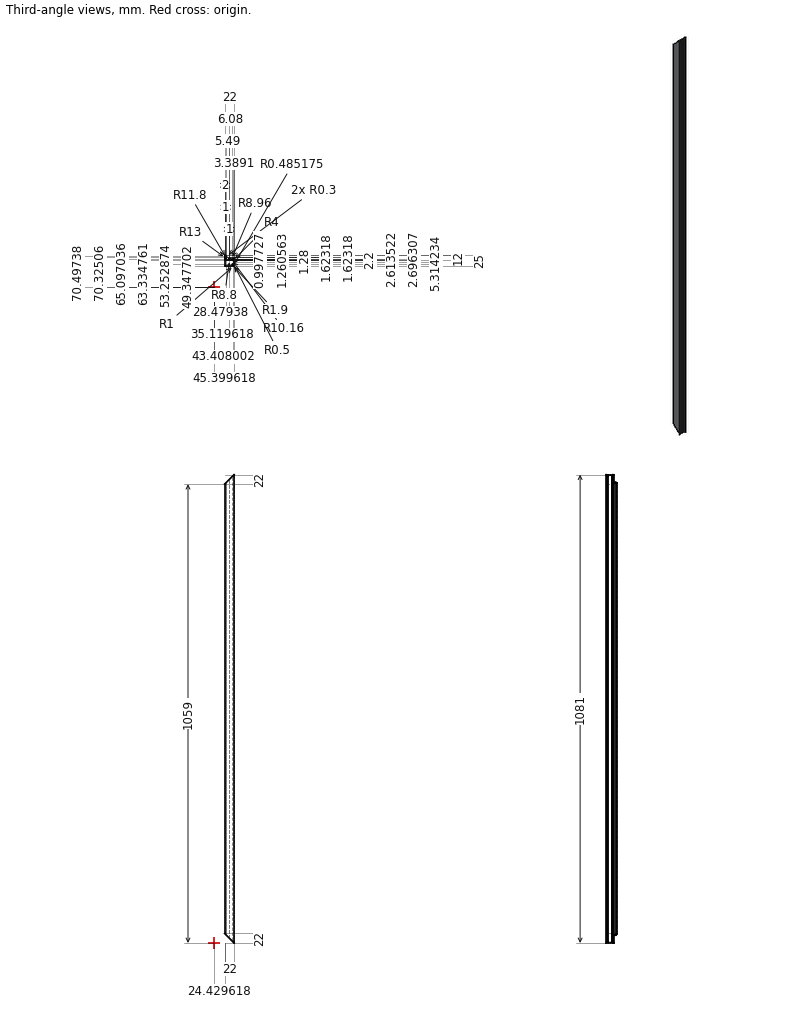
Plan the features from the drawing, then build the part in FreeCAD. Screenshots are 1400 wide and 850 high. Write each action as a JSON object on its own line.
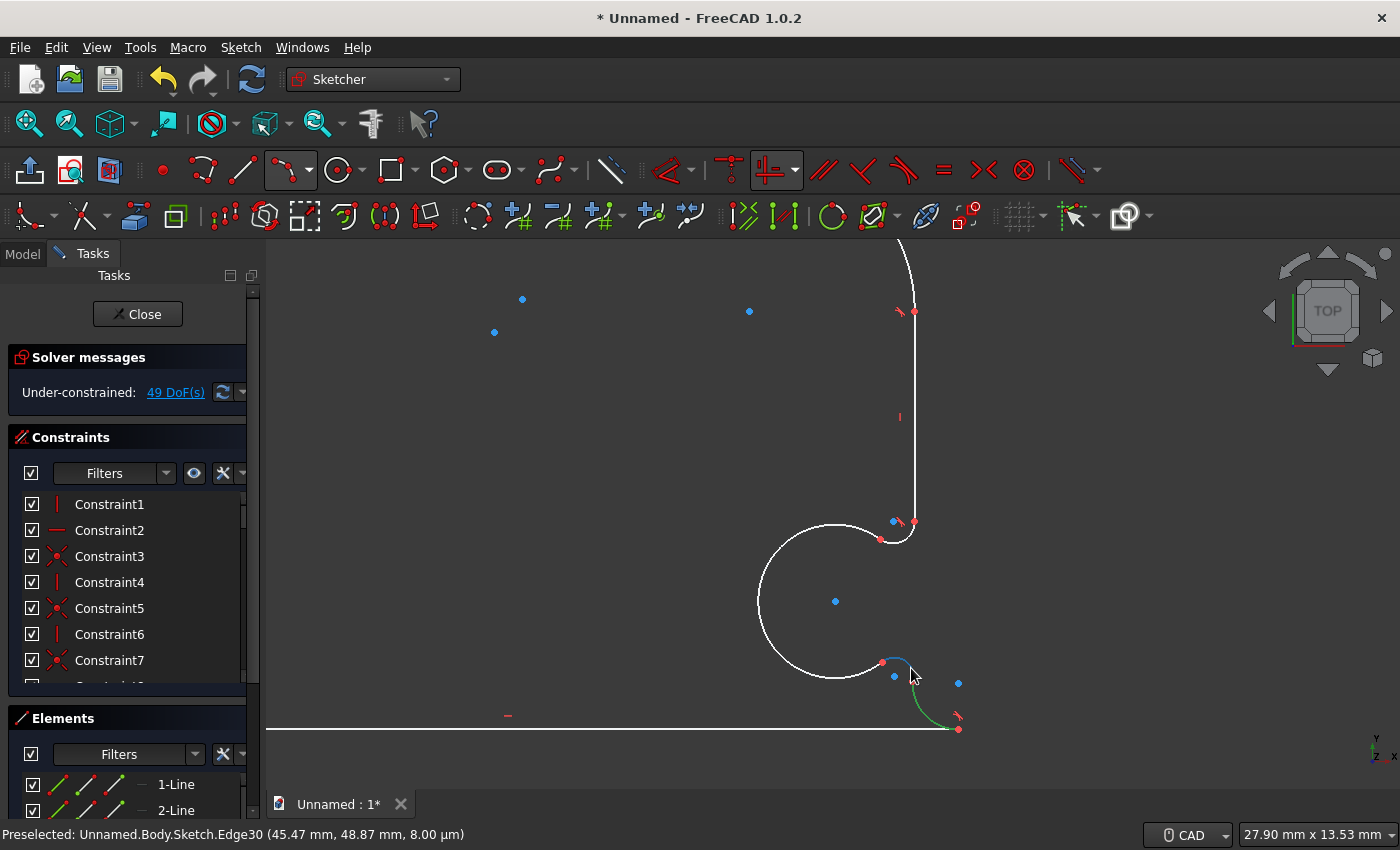
{"action": "left_click", "coordinate": [911, 667]}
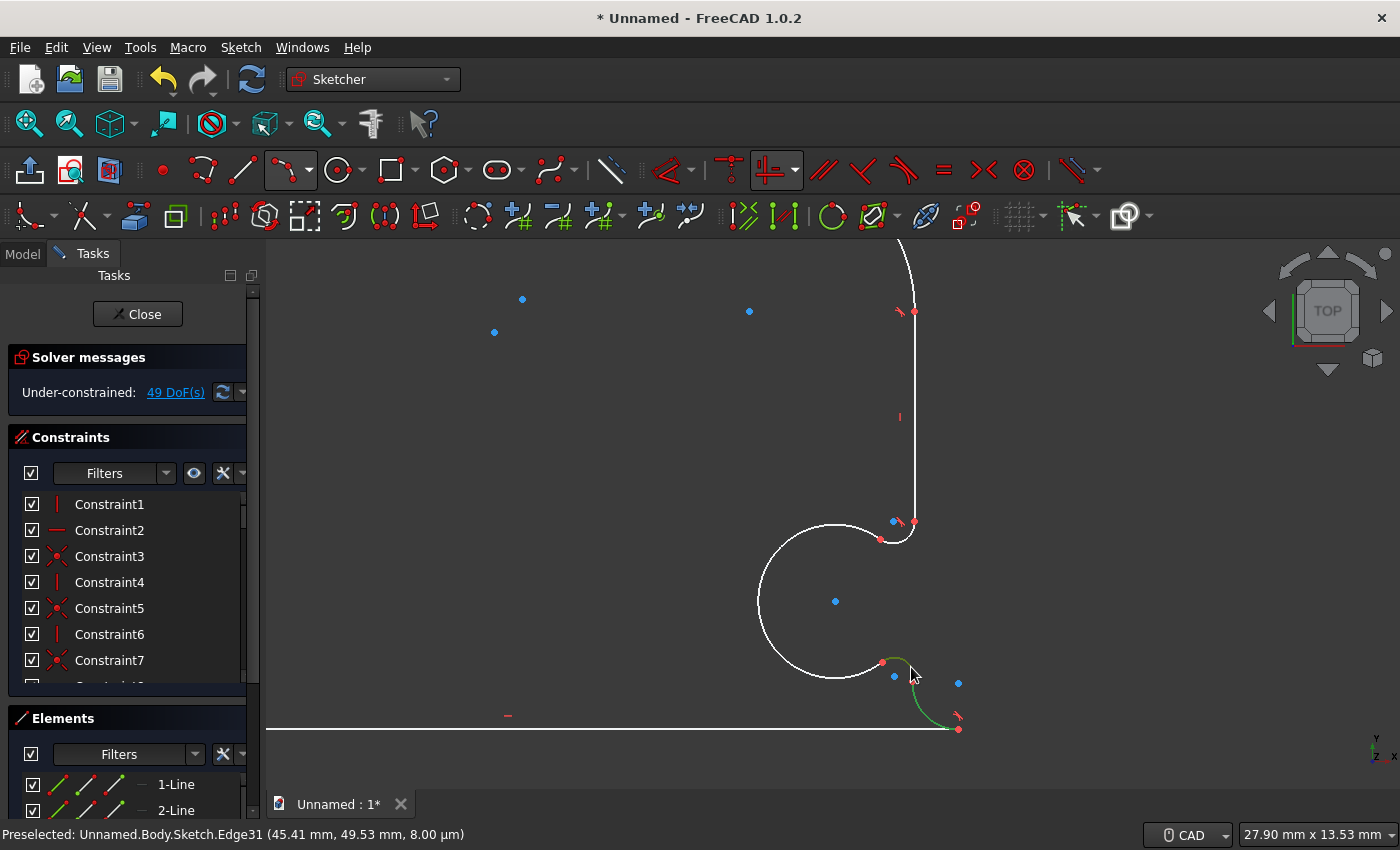
{"action": "left_click", "coordinate": [904, 170]}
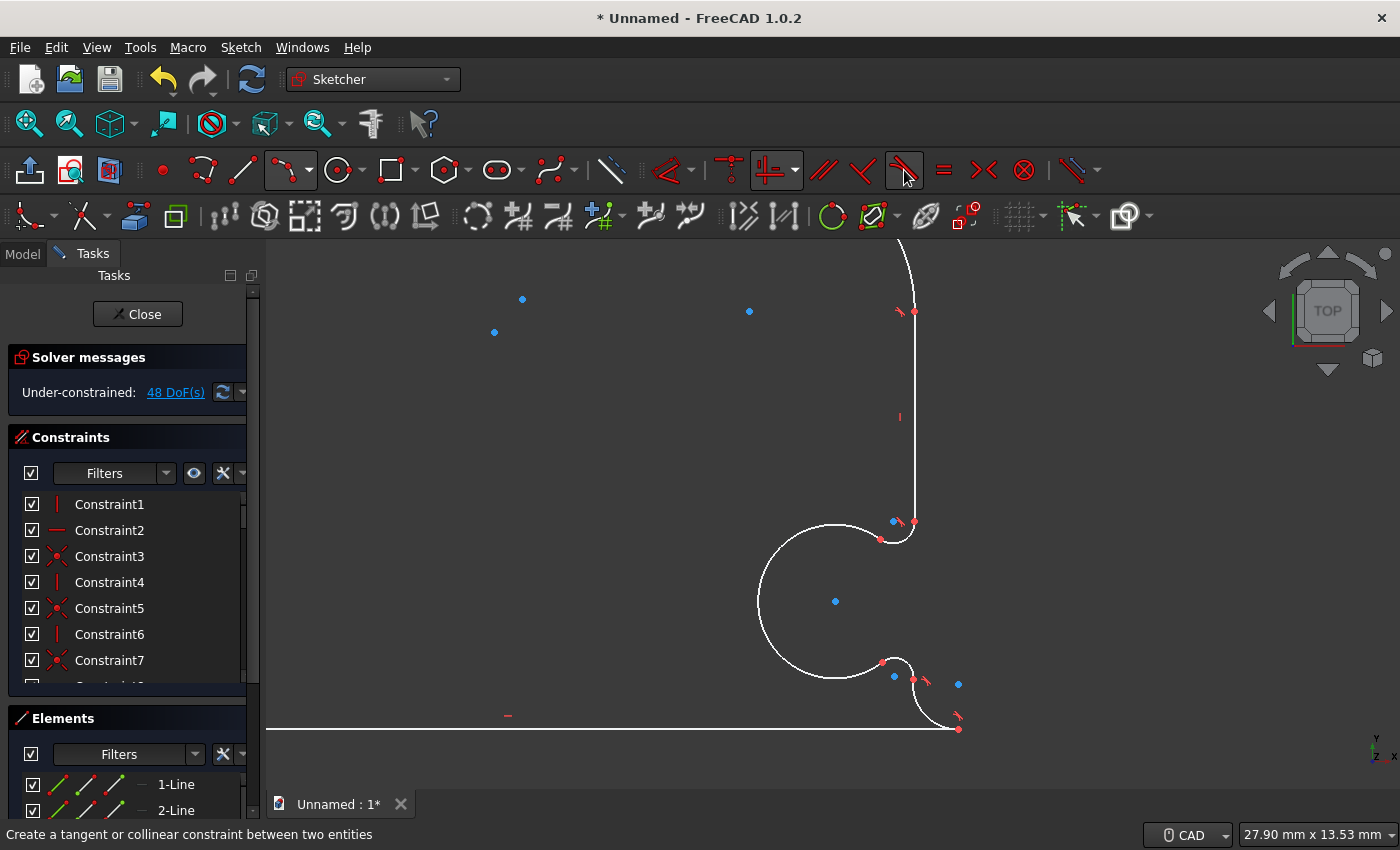
{"action": "left_click", "coordinate": [910, 666]}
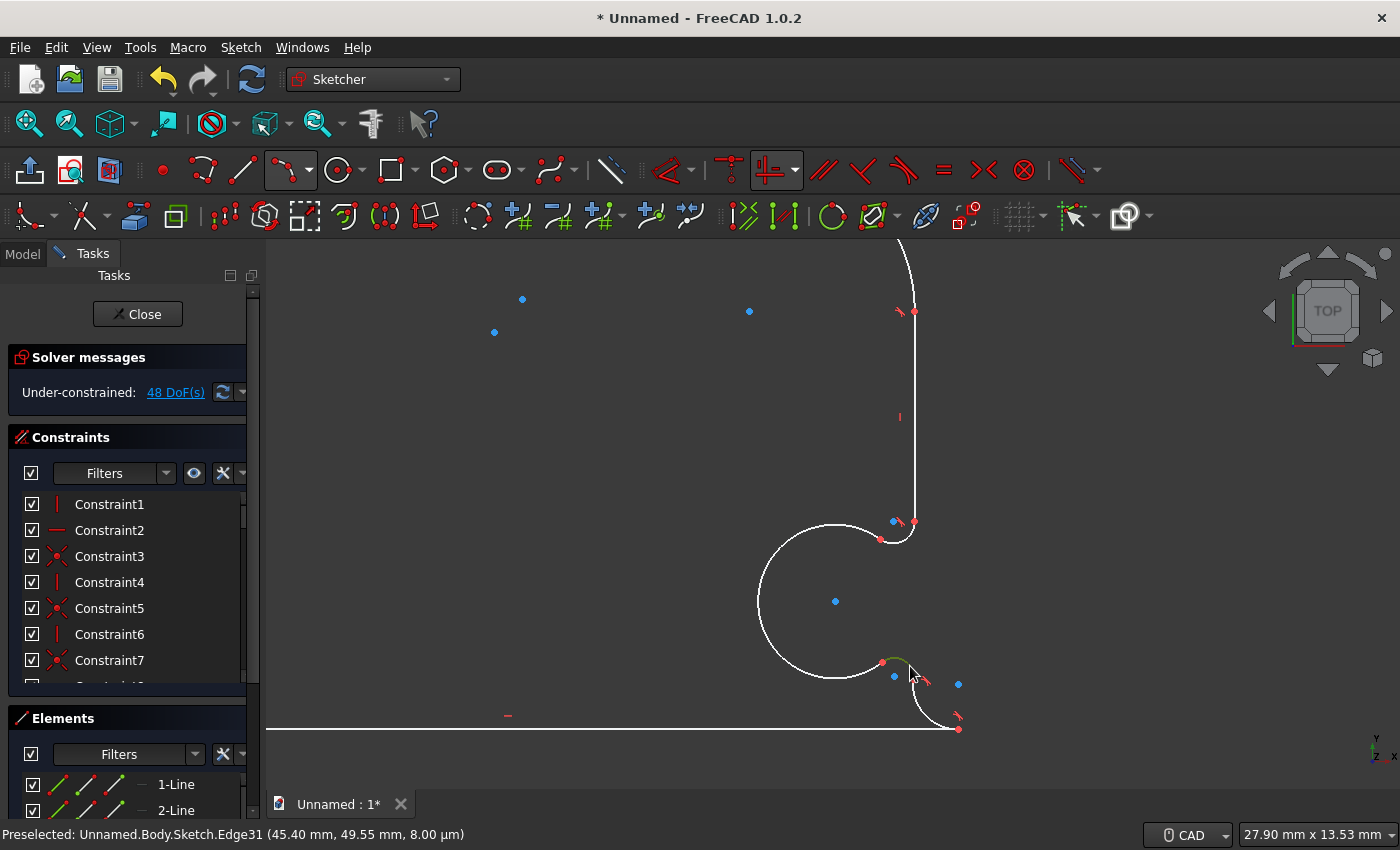
{"action": "left_click", "coordinate": [786, 543]}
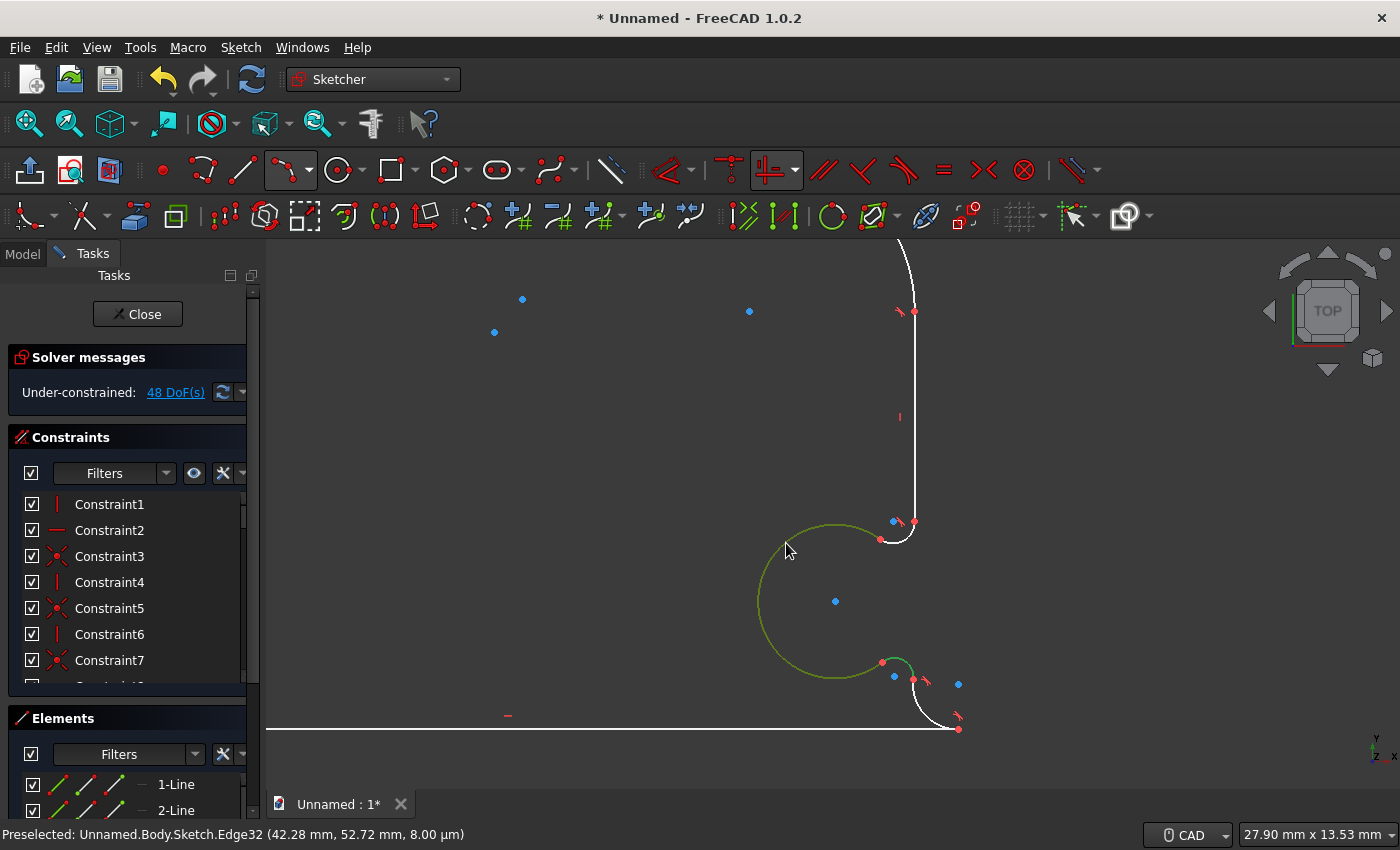
{"action": "left_click", "coordinate": [904, 170]}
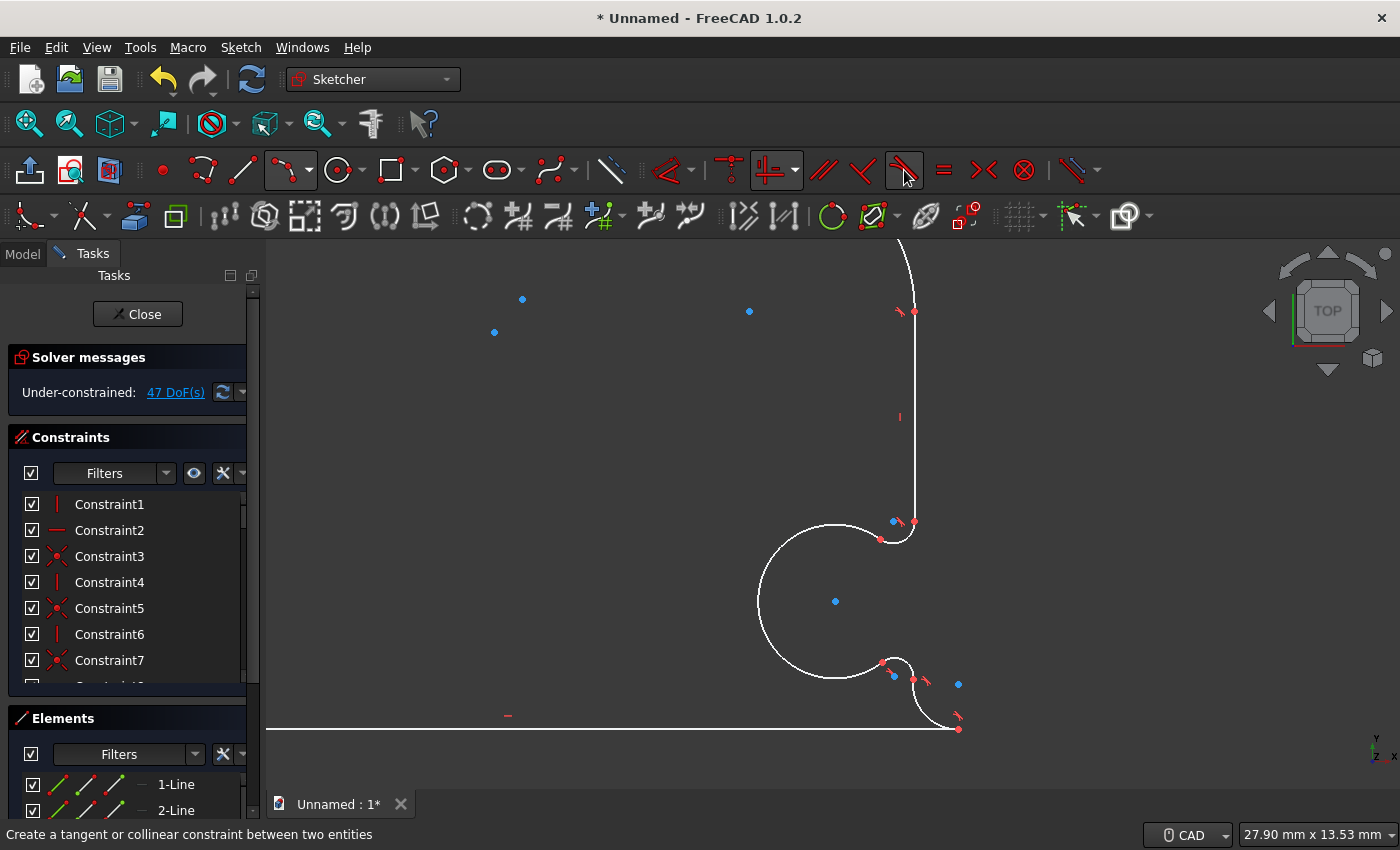
{"action": "left_click", "coordinate": [786, 543]}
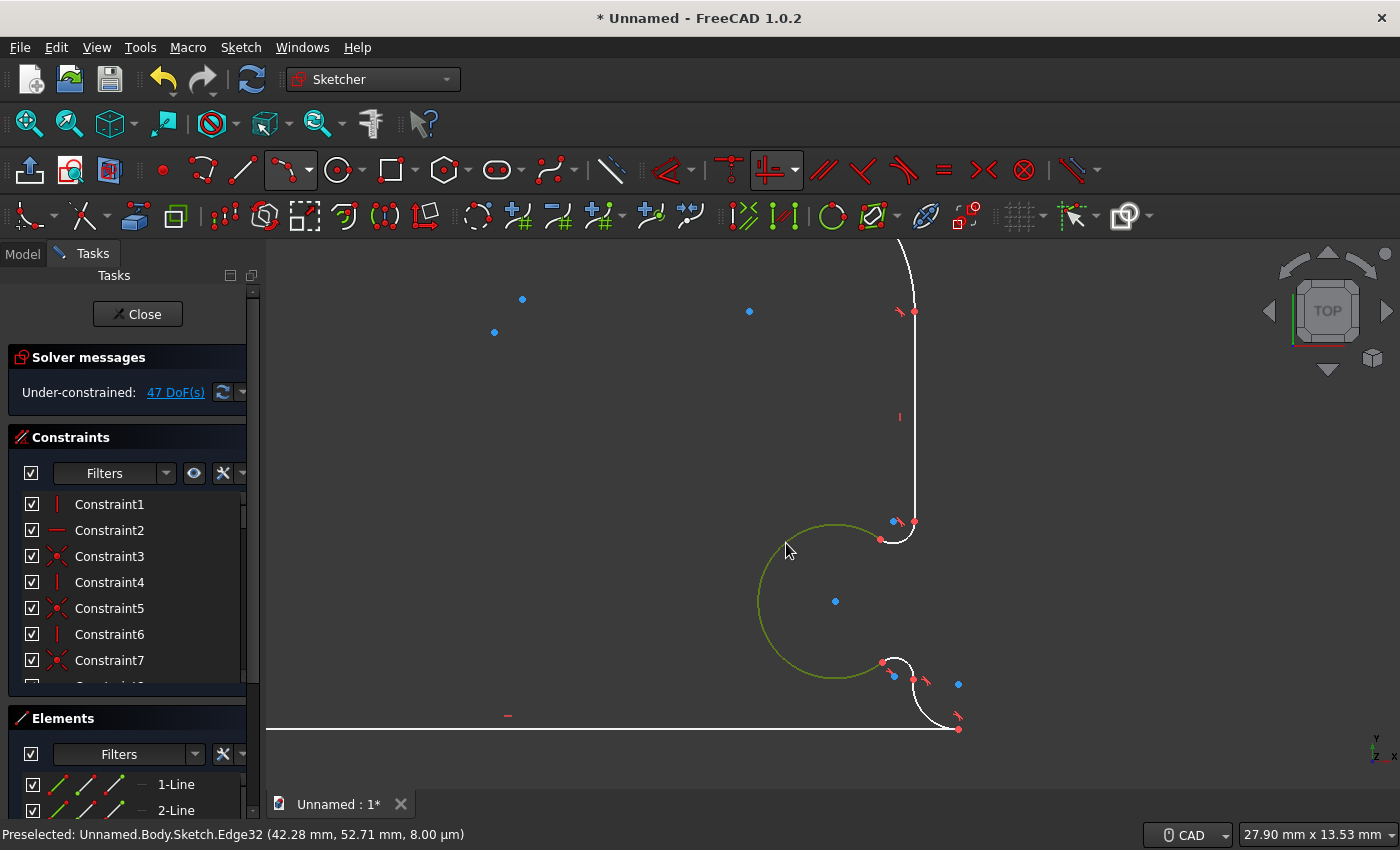
{"action": "left_click", "coordinate": [894, 543]}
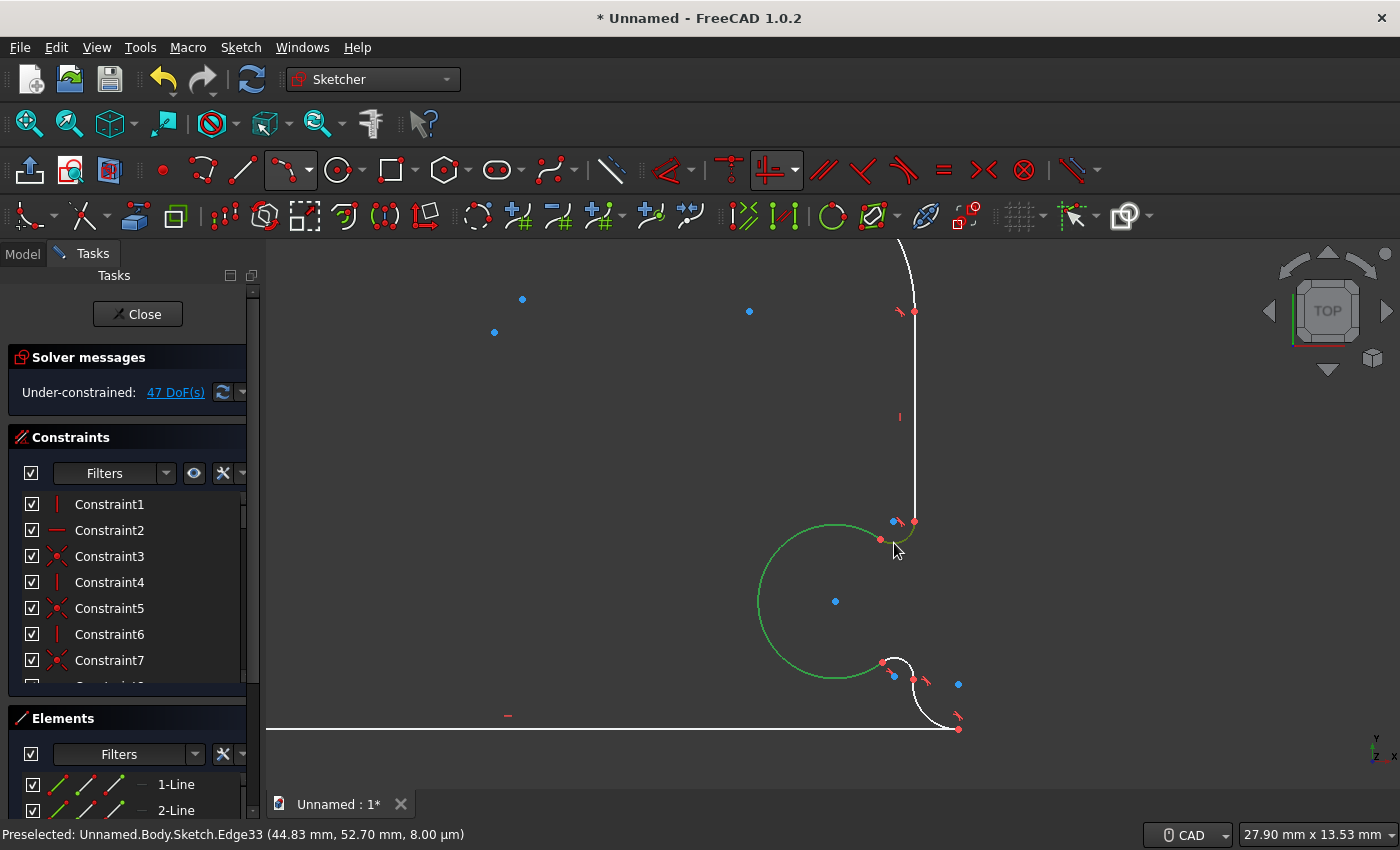
{"action": "left_click", "coordinate": [904, 170]}